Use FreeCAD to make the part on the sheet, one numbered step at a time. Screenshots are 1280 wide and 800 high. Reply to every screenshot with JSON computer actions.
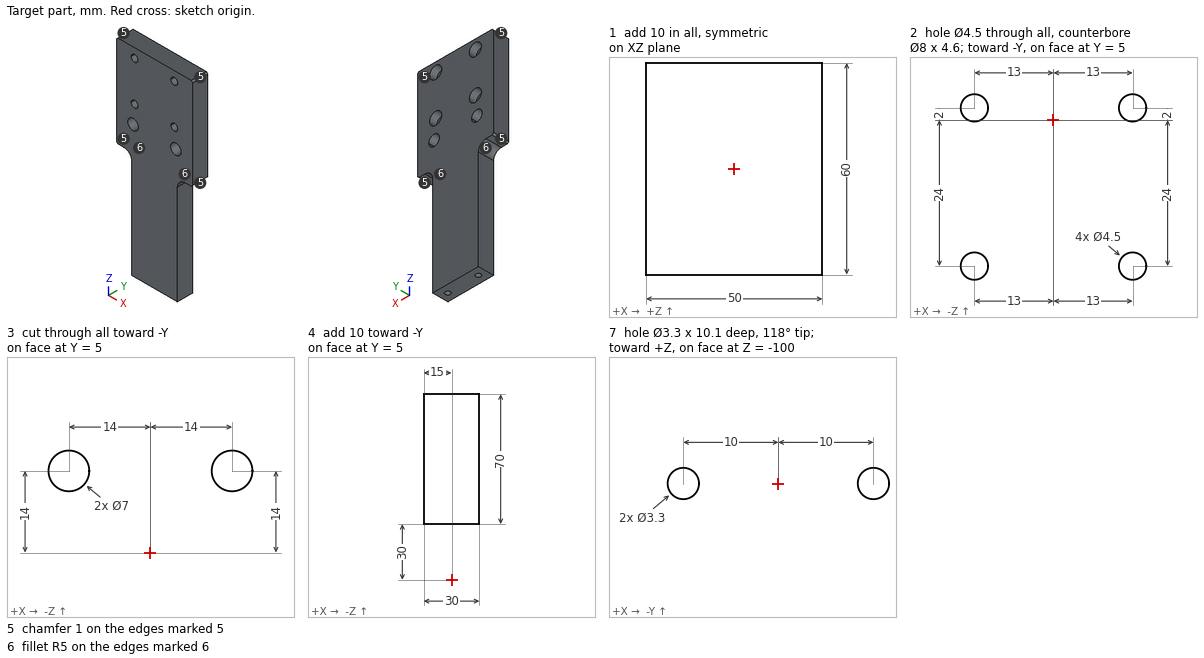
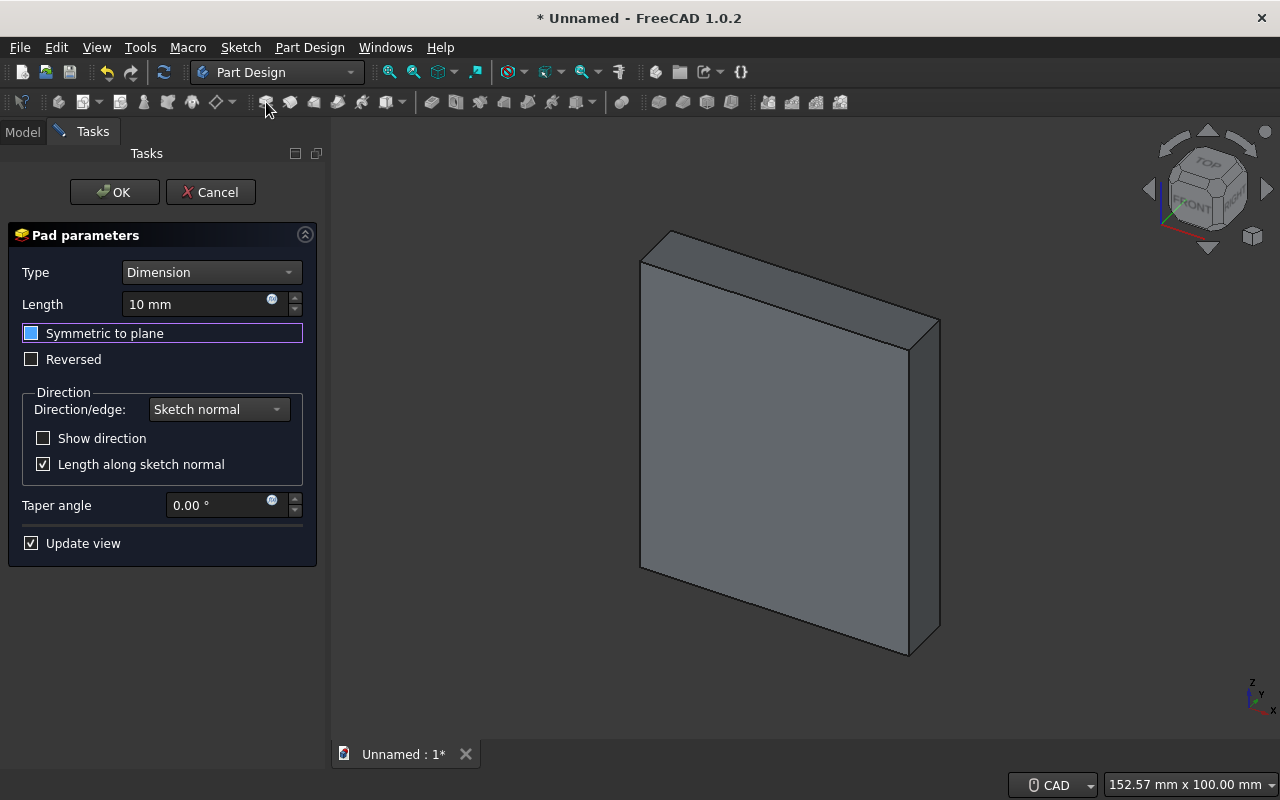
{"action": "left_click", "coordinate": [30, 333]}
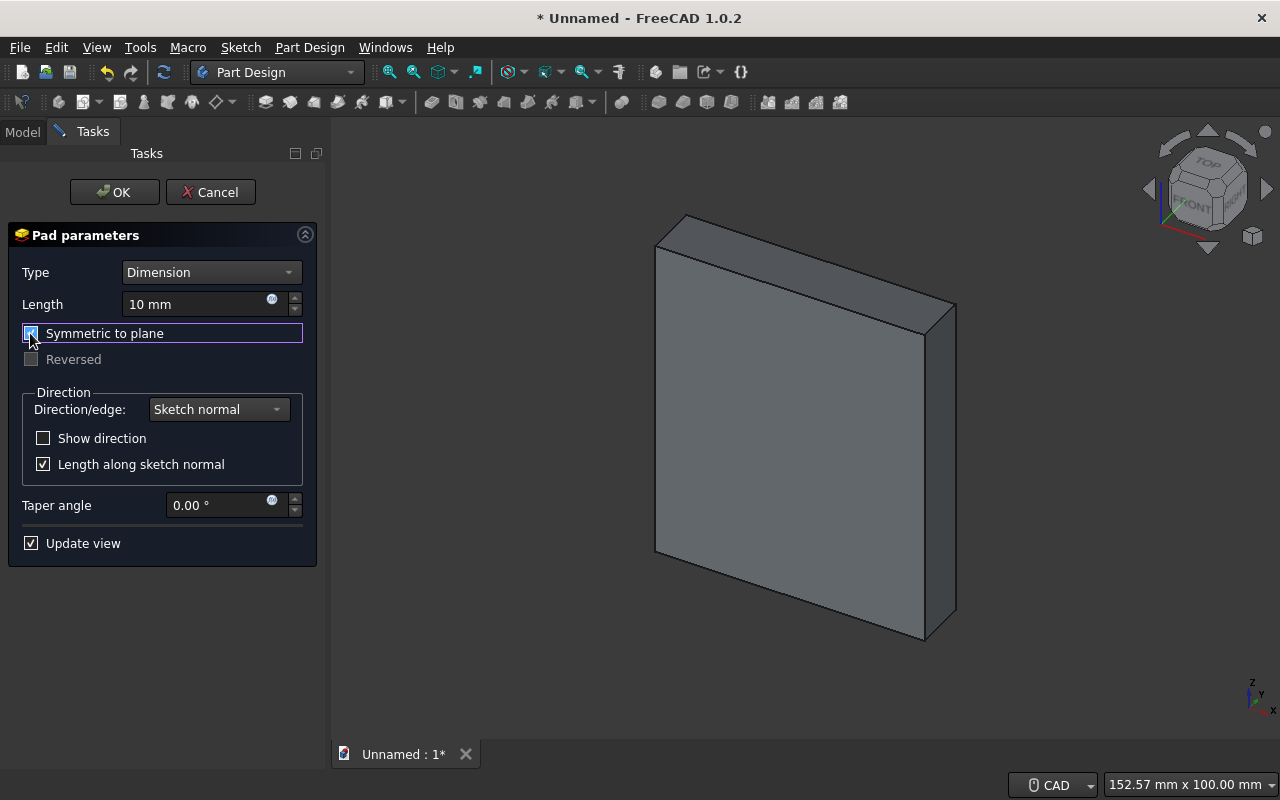
{"action": "left_click", "coordinate": [115, 192]}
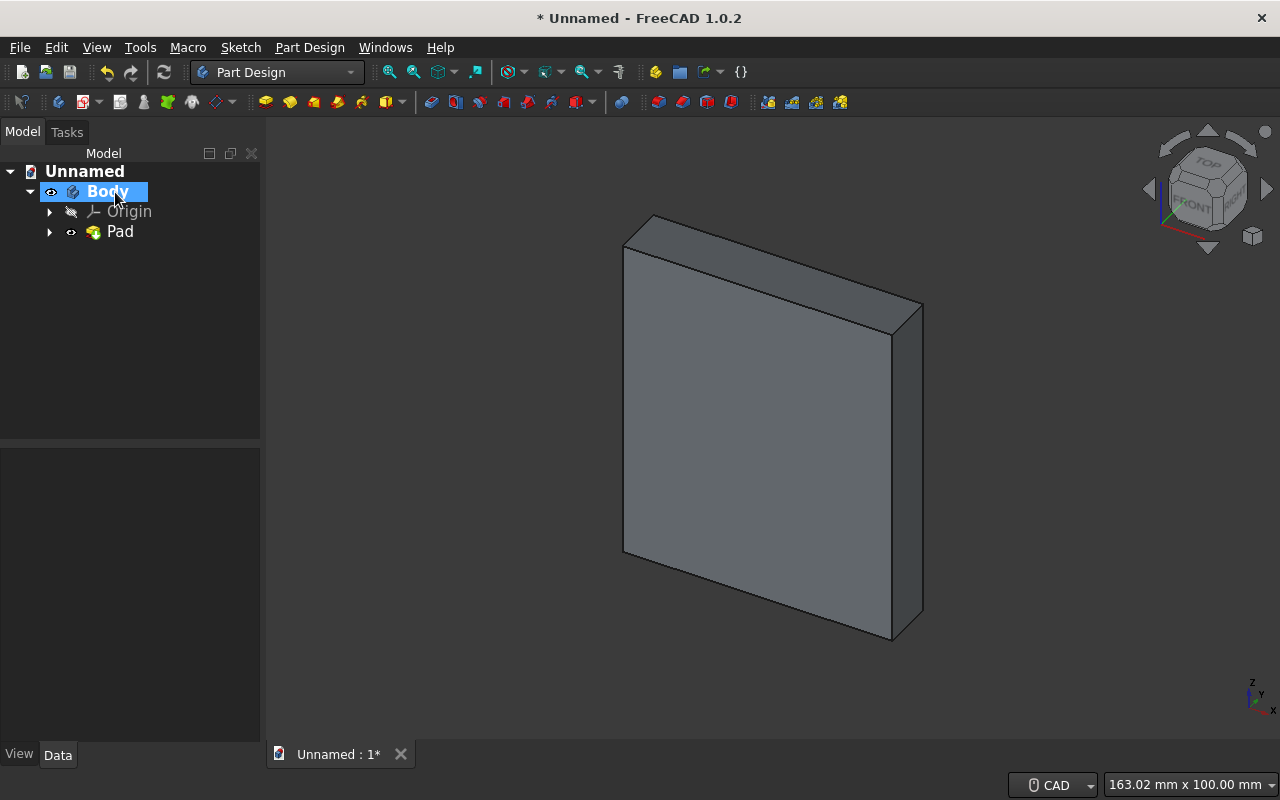
{"action": "key", "text": "4"}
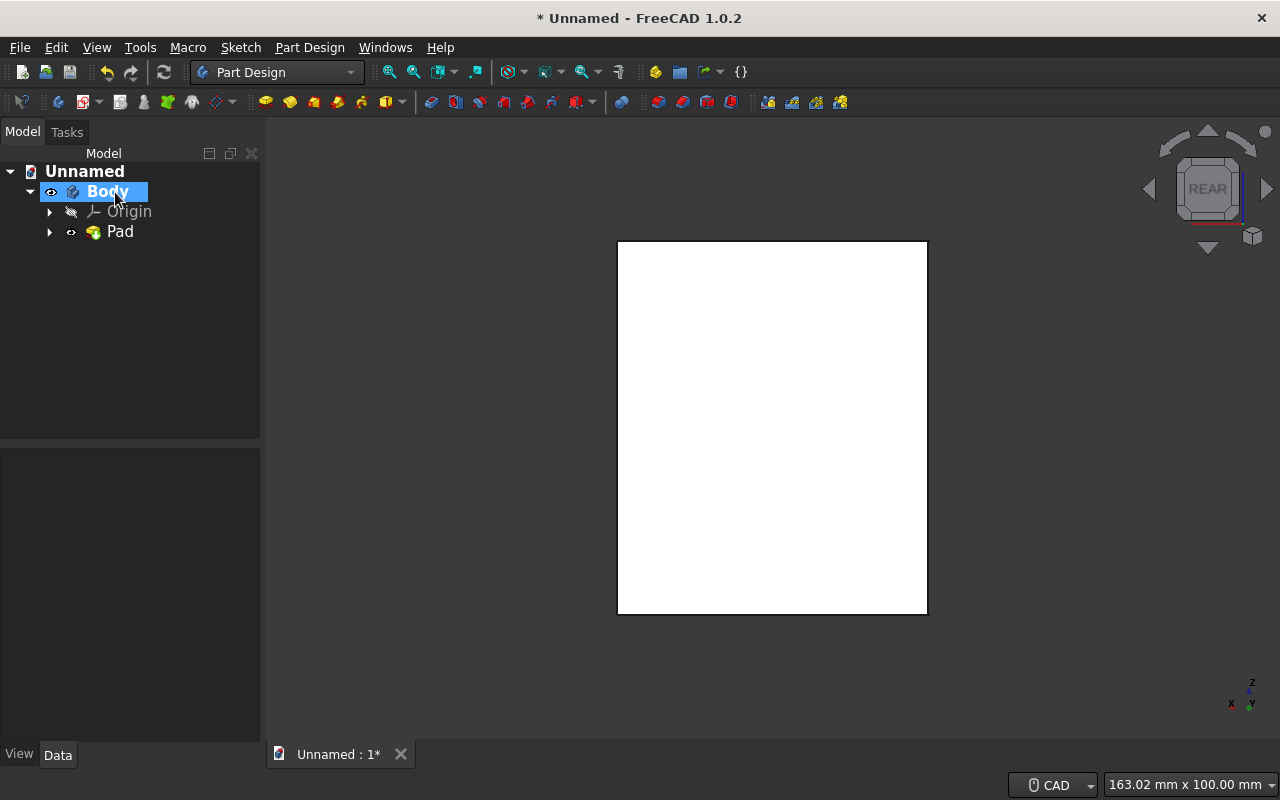
{"action": "left_click", "coordinate": [773, 427]}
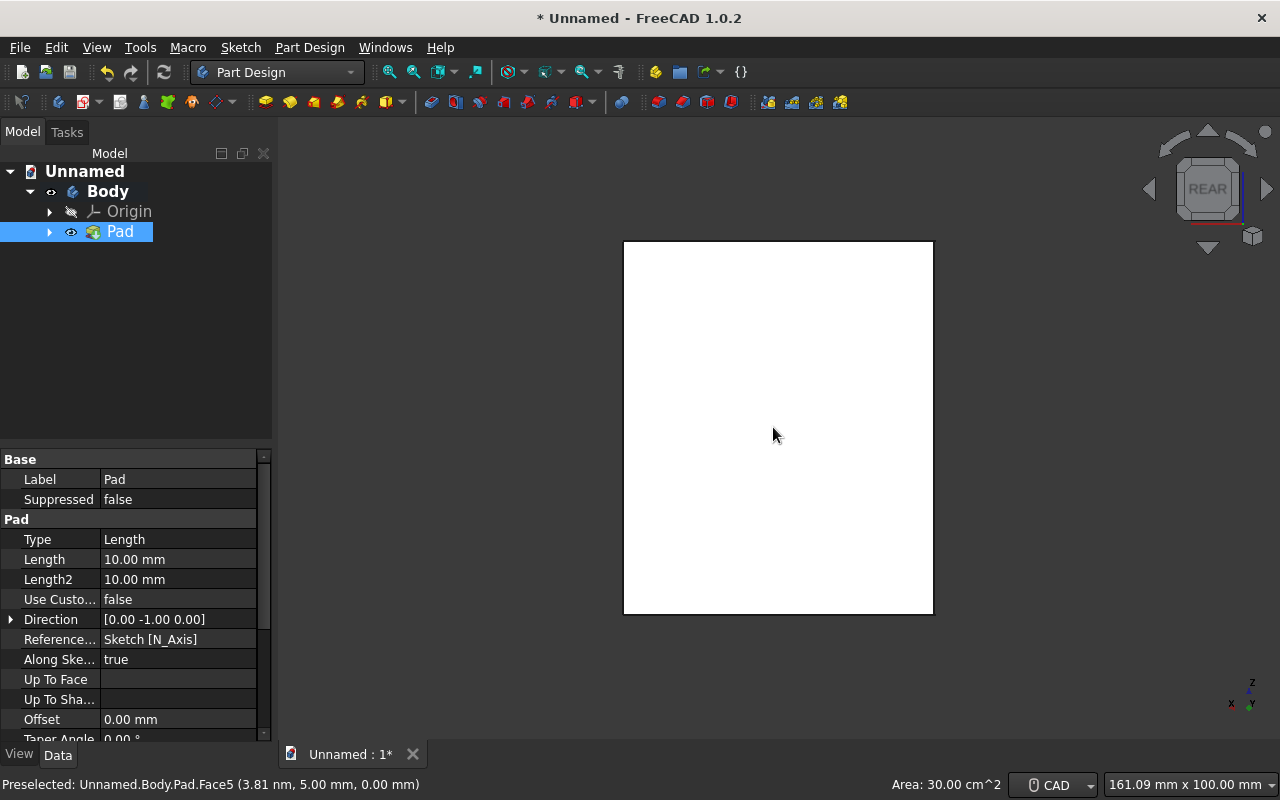
{"action": "left_click", "coordinate": [84, 102]}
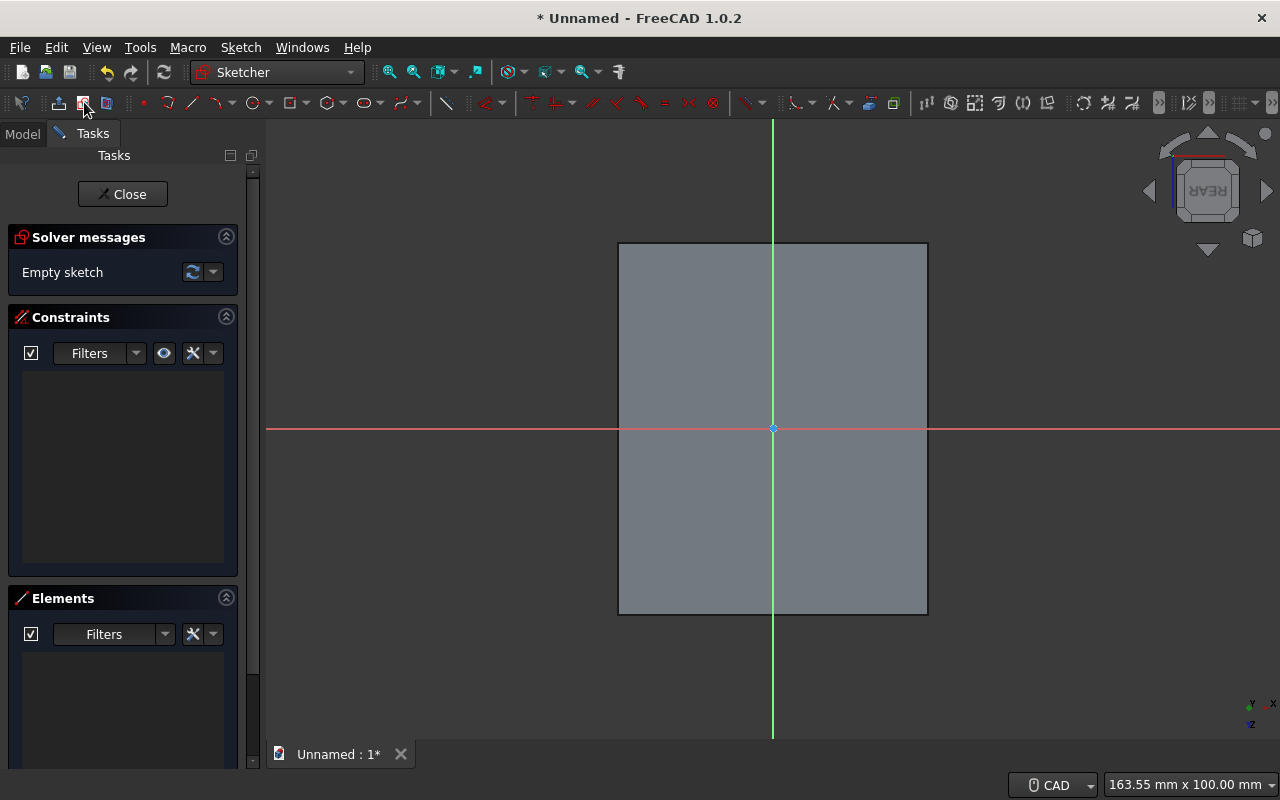
{"action": "scroll", "coordinate": [829, 553], "scroll_direction": "up", "scroll_amount": 4}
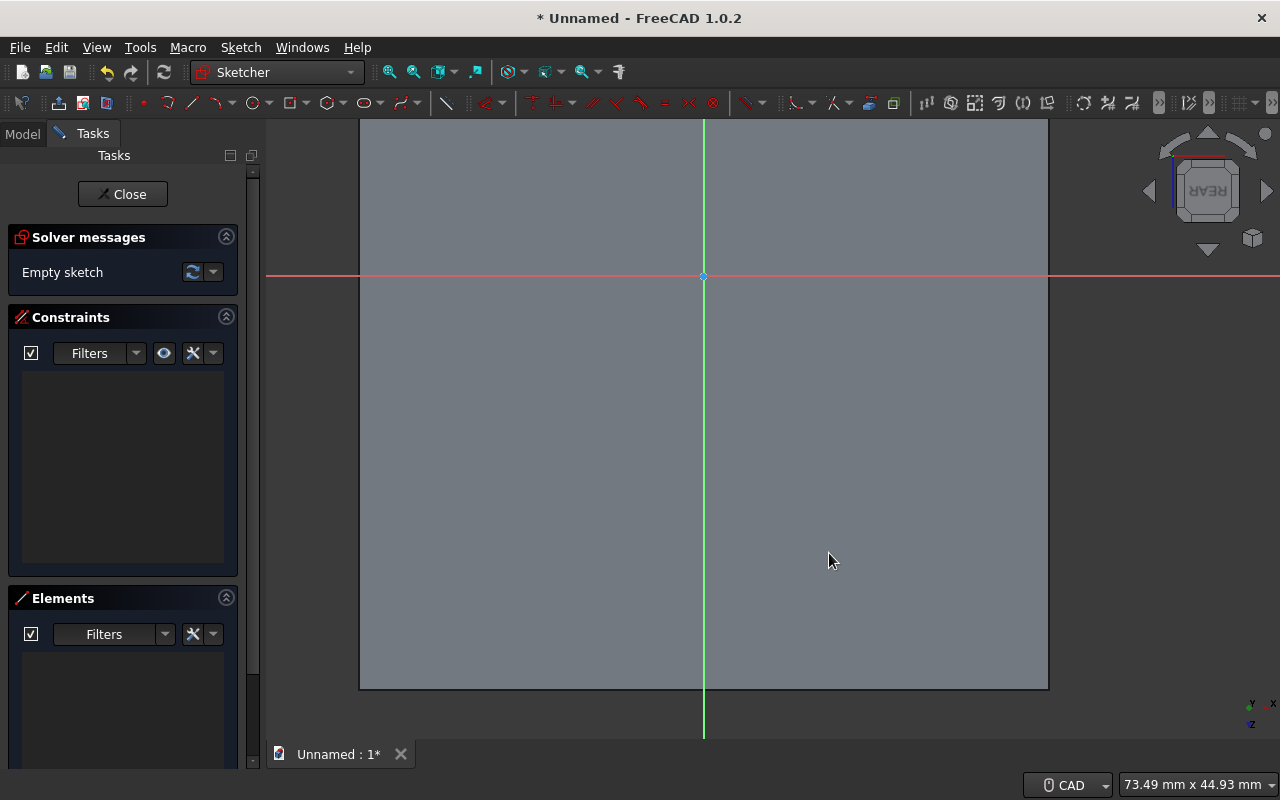
{"action": "left_click", "coordinate": [254, 104]}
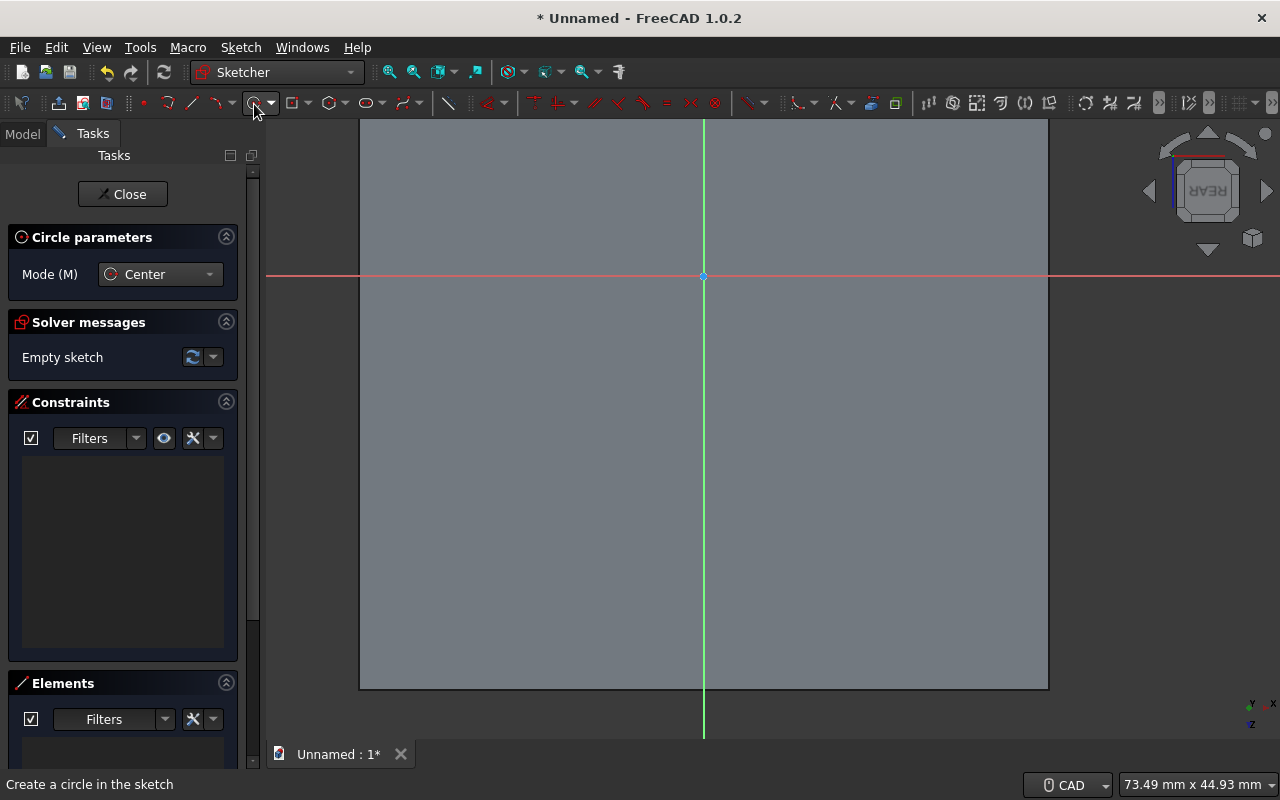
{"action": "left_click", "coordinate": [883, 607]}
{"action": "mouse_move", "coordinate": [905, 585]}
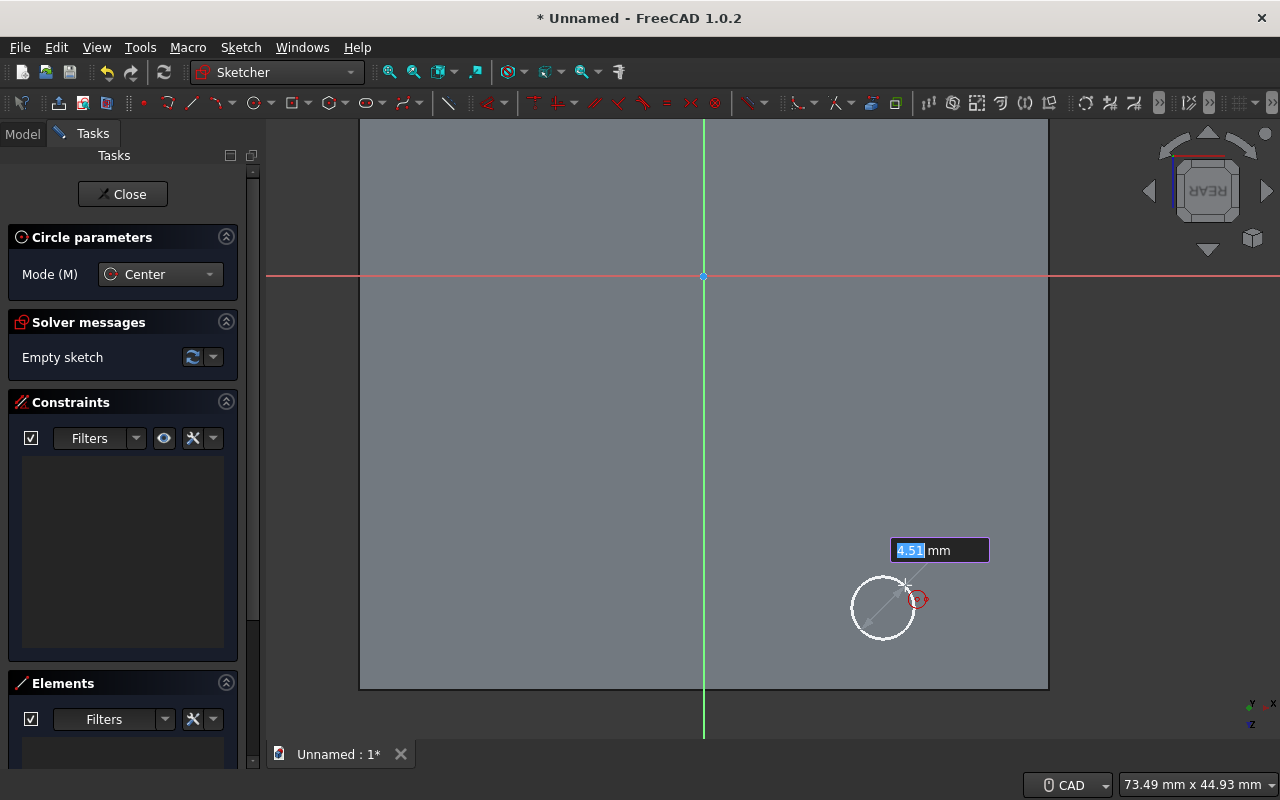
{"action": "type", "text": "4.5"}
{"action": "key", "text": "Return"}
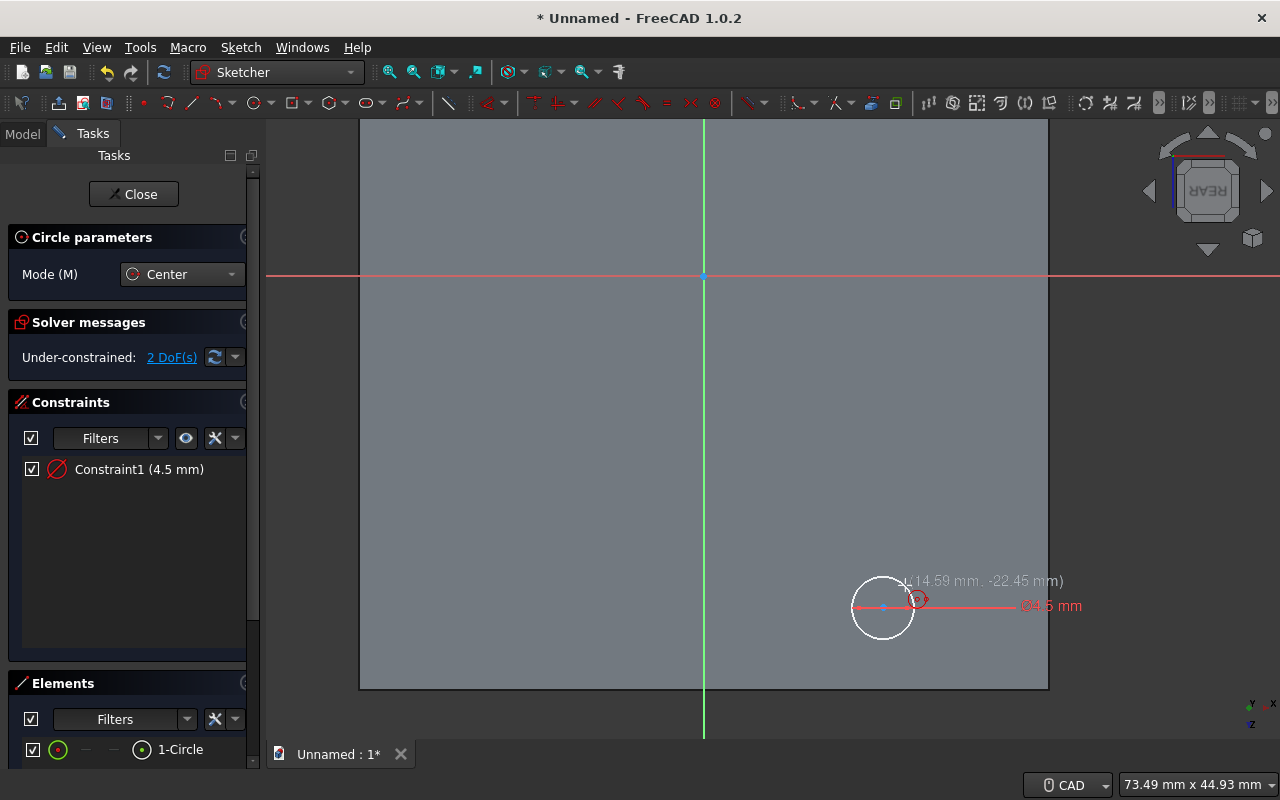
{"action": "left_click", "coordinate": [883, 249]}
{"action": "mouse_move", "coordinate": [905, 227]}